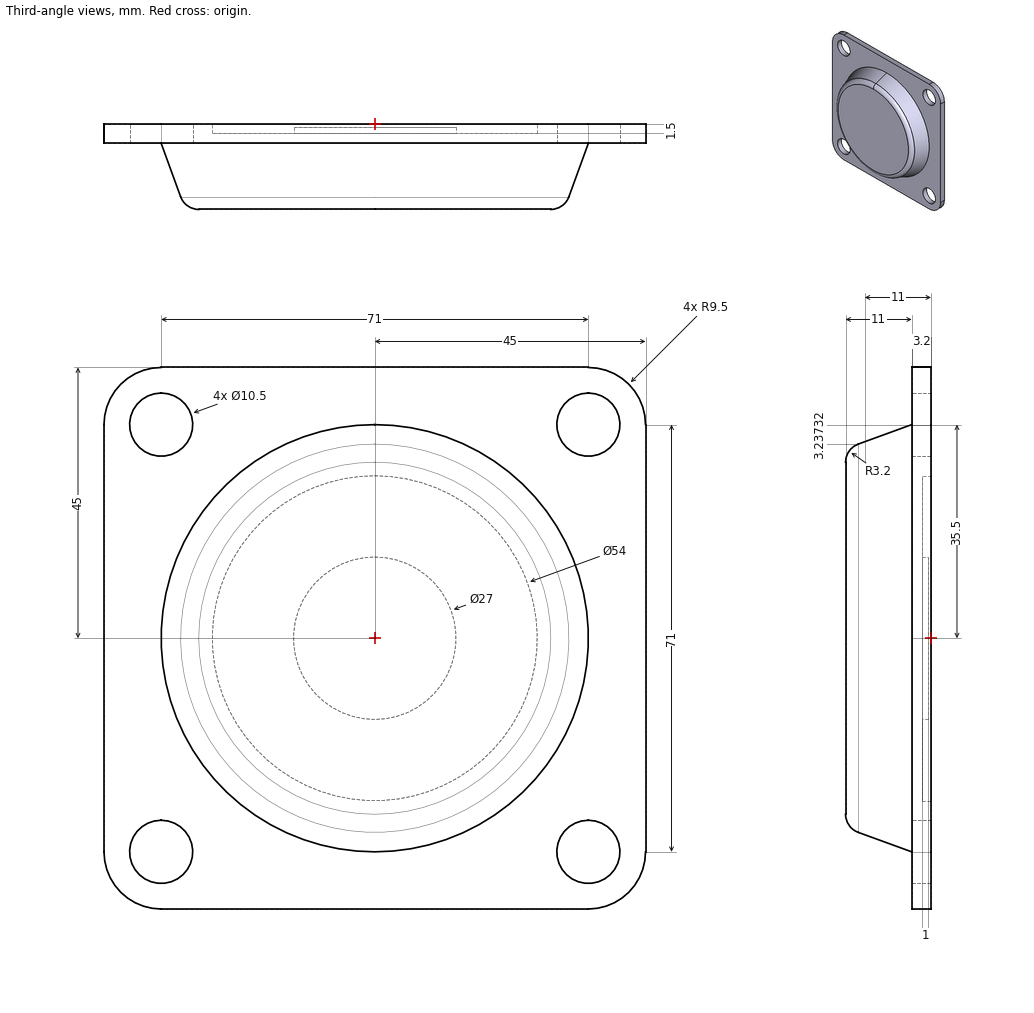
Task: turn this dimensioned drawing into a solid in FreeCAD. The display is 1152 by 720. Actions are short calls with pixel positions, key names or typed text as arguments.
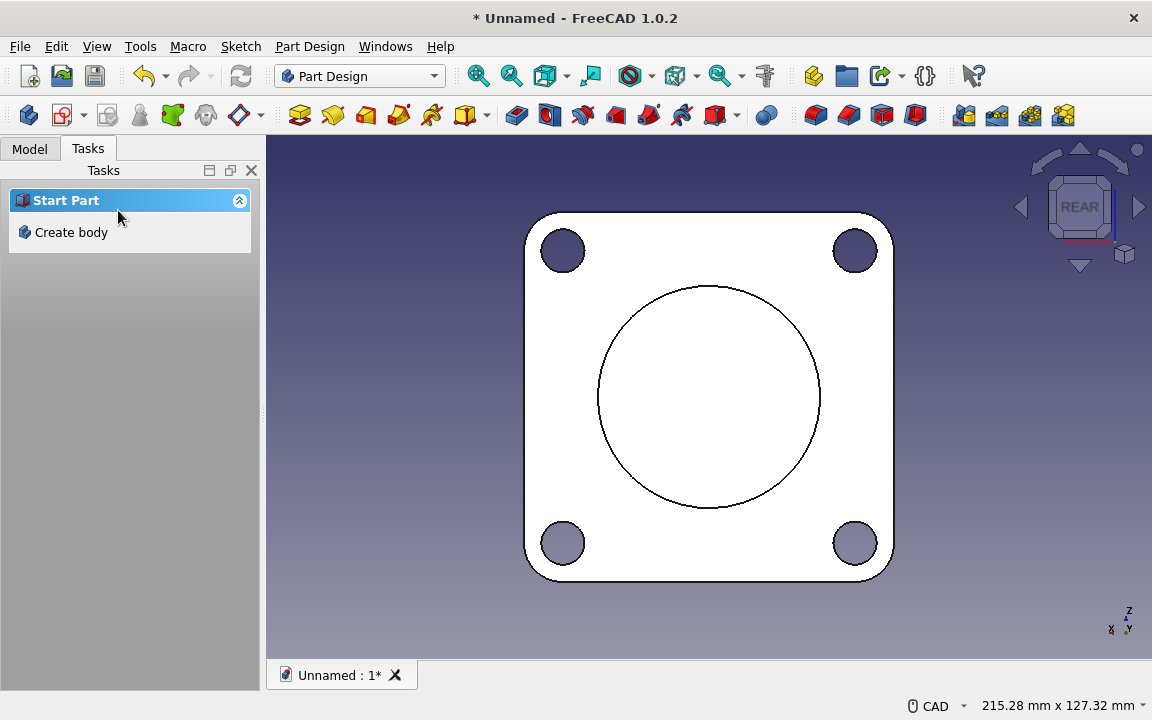
click(709, 396)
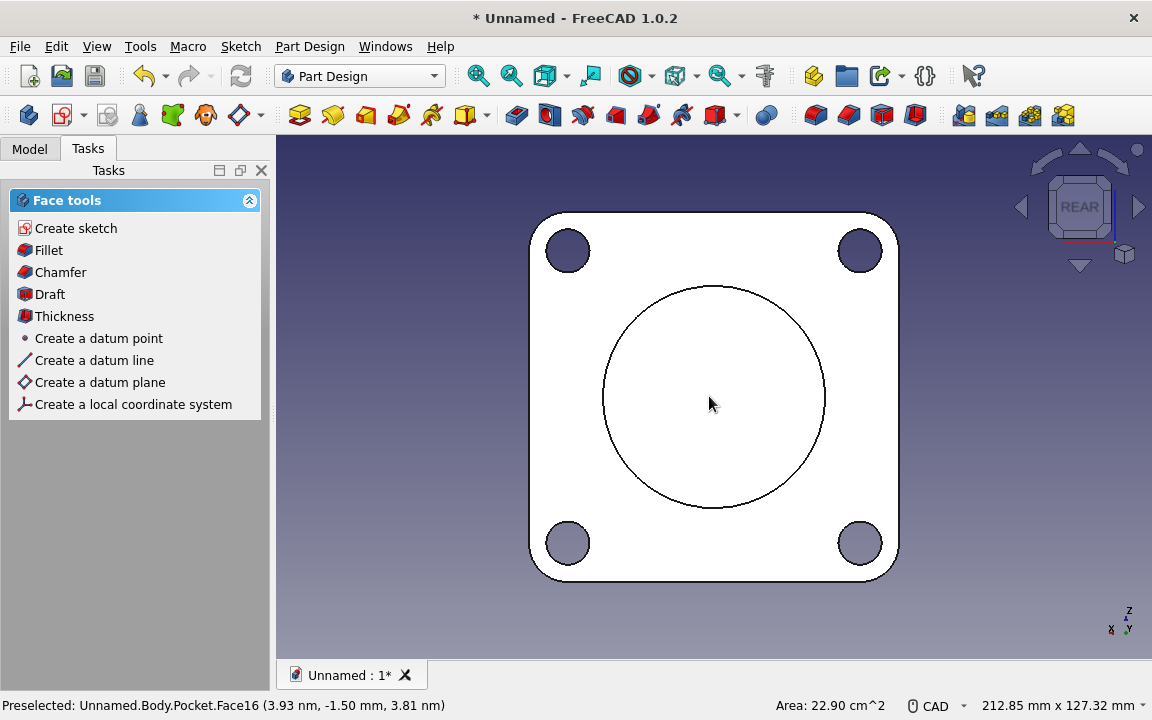
click(62, 116)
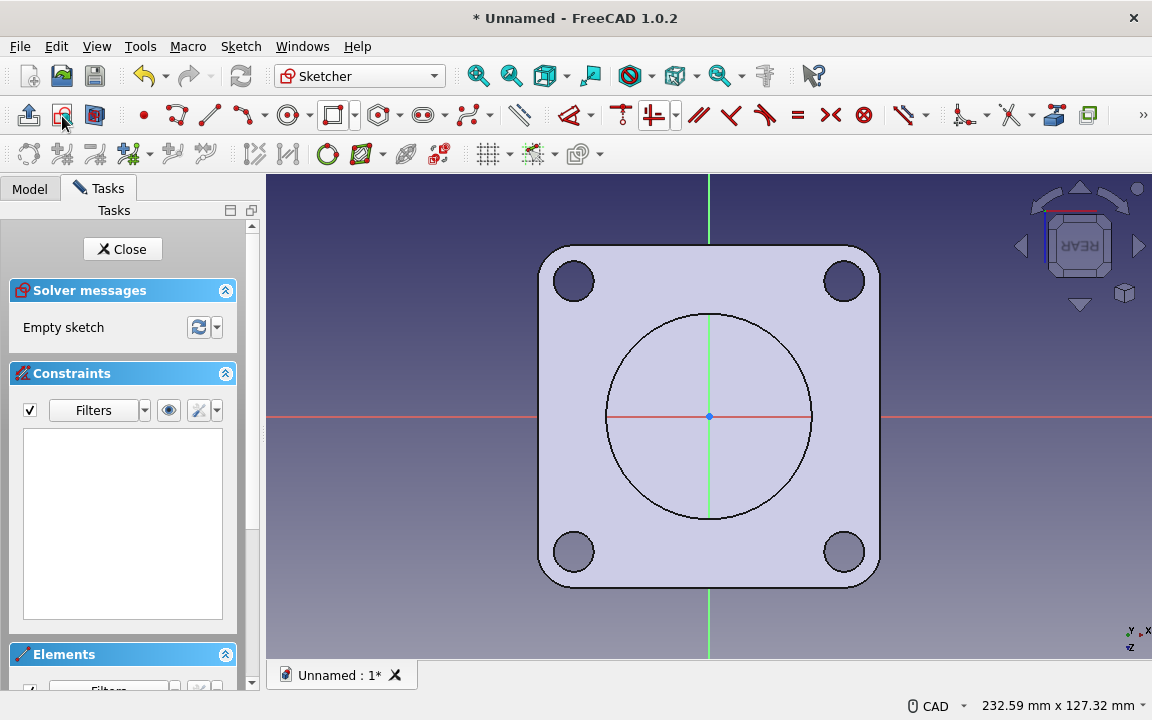
key(q)
key(s)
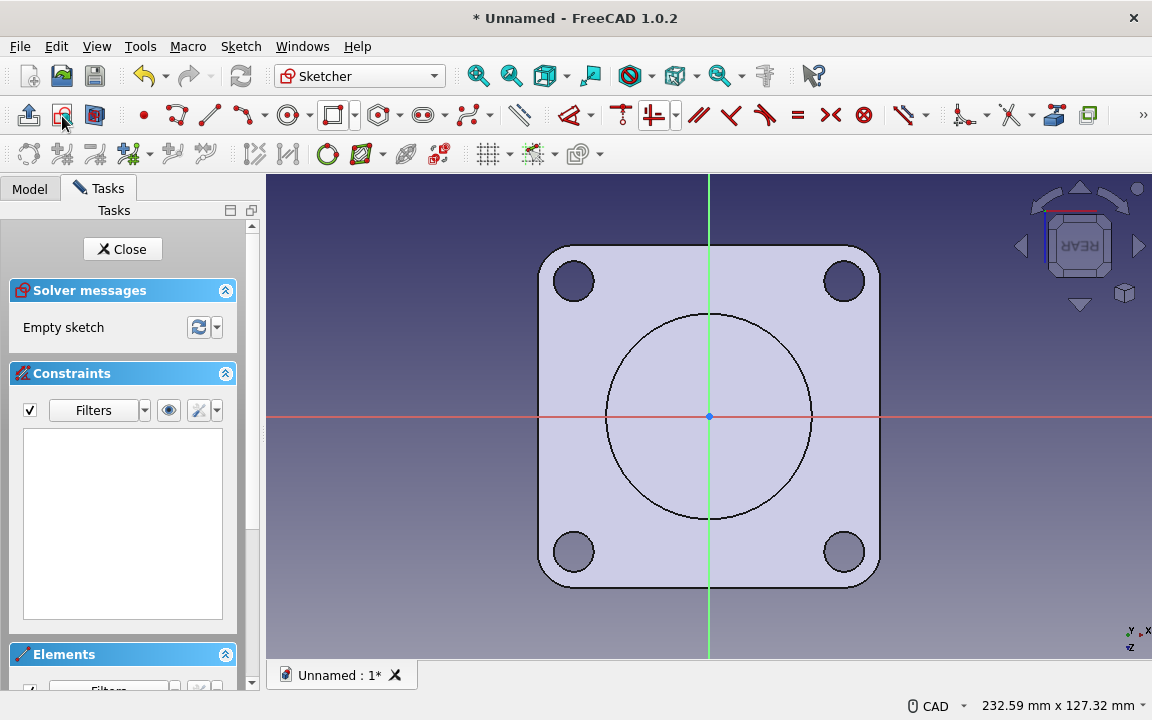
scroll(749, 416, up, 5)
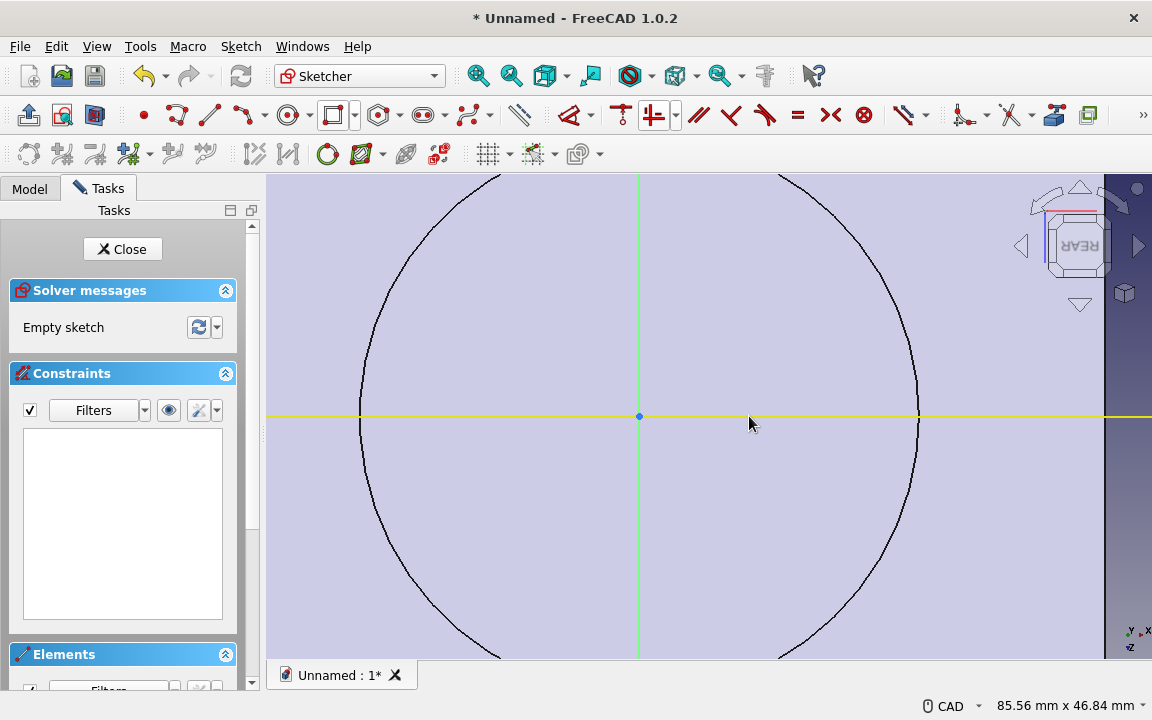
key(g)
key(c)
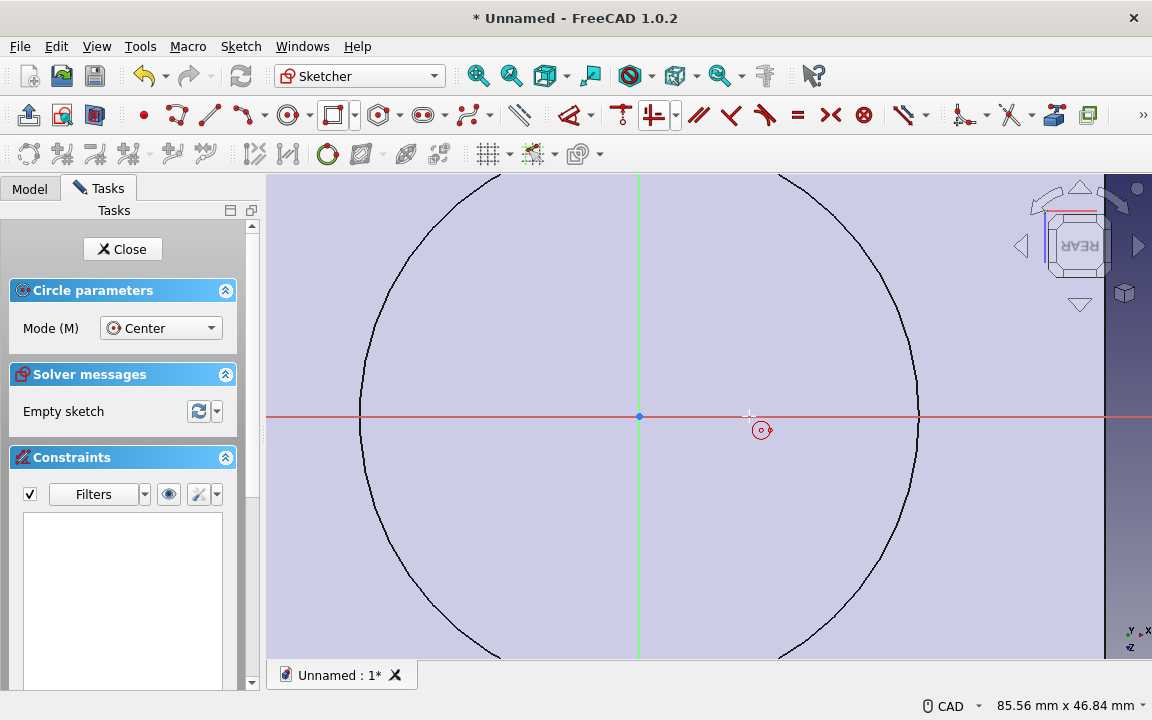
click(639, 416)
move(738, 318)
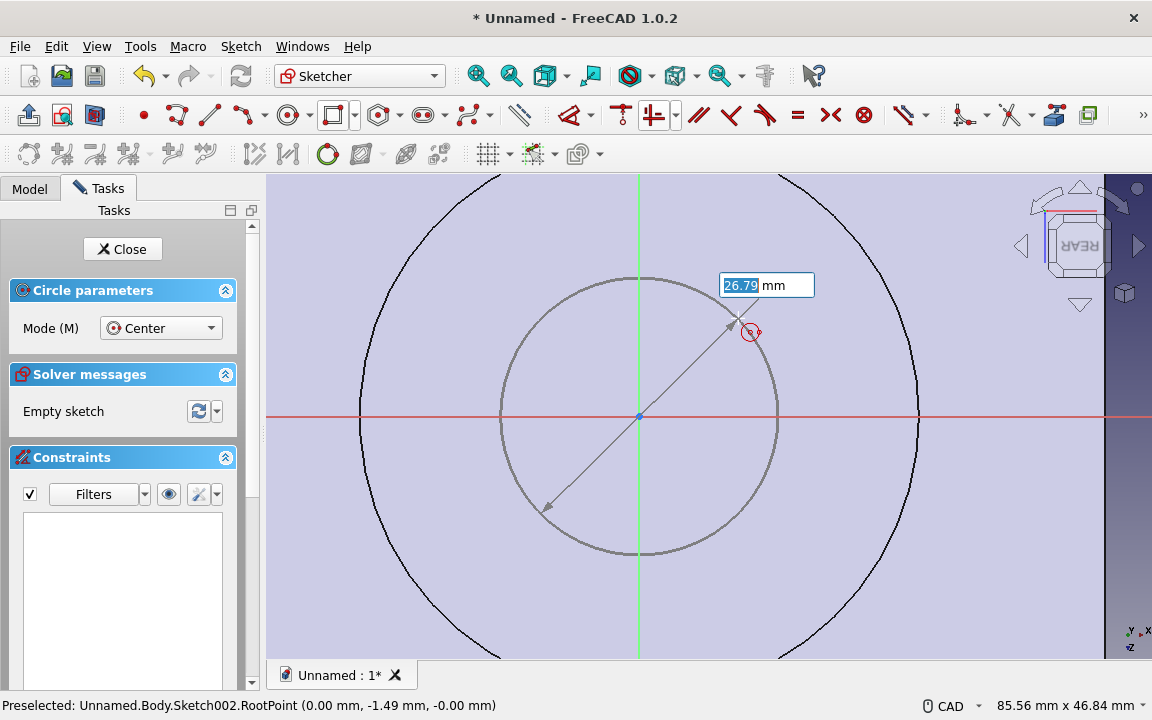
text(27)
key(Return)
key(Escape)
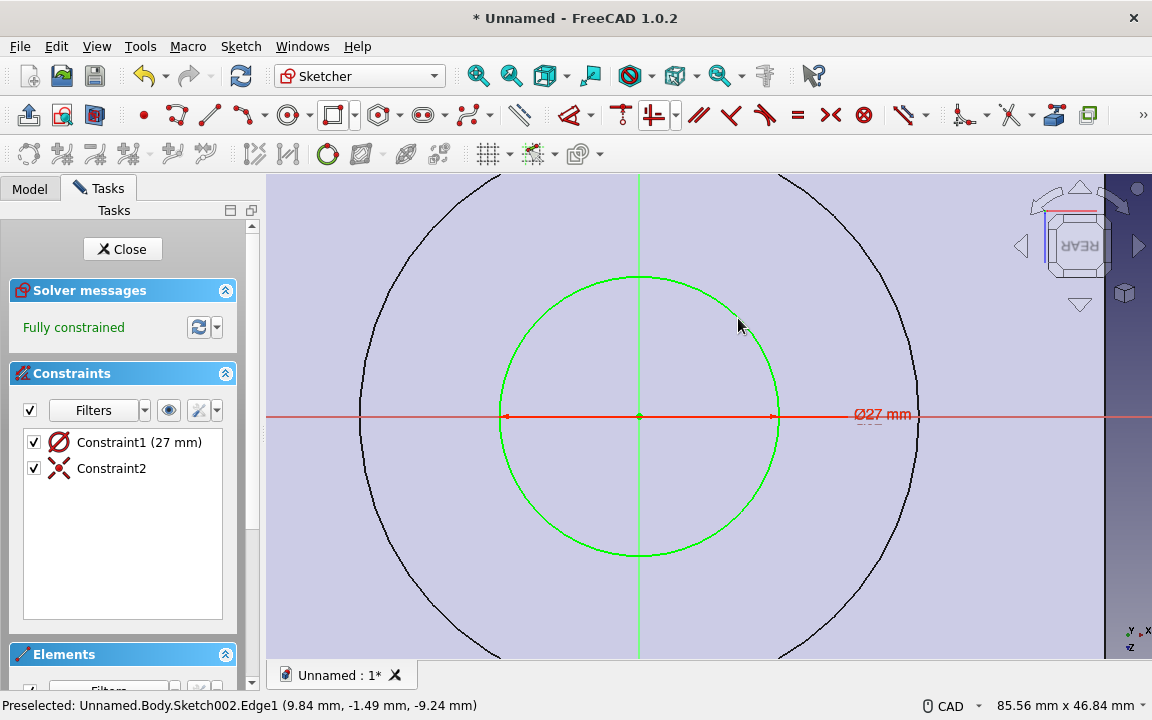
click(123, 249)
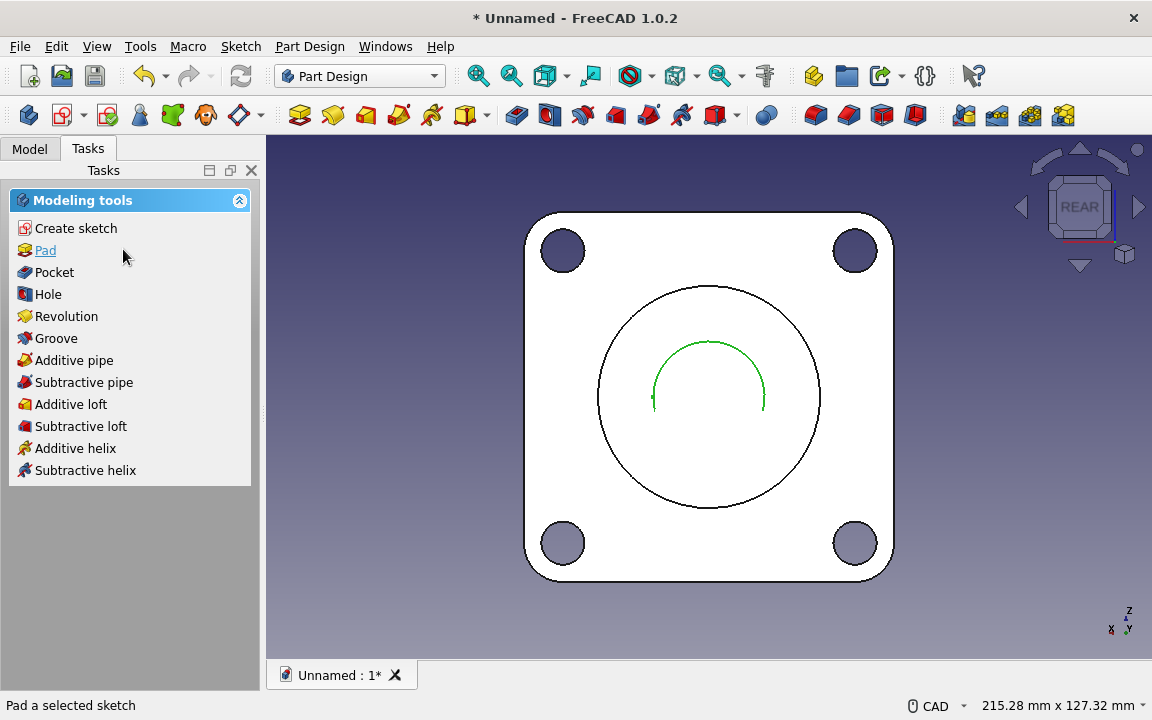
click(300, 116)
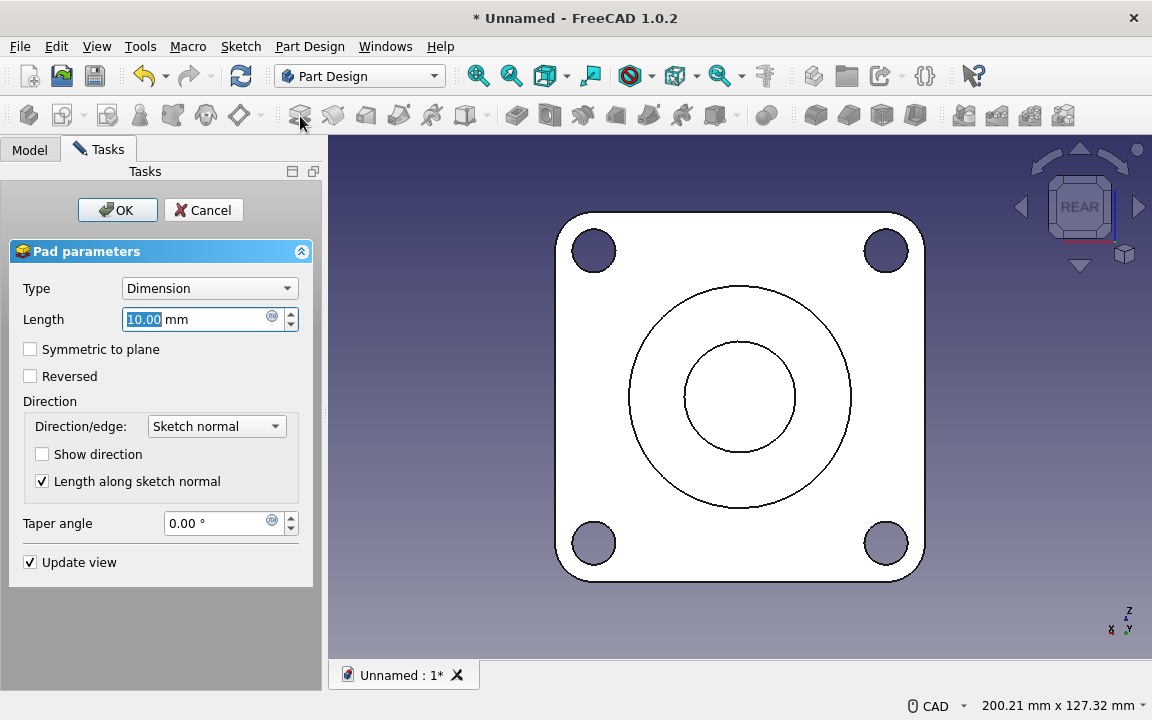
text(1)
key(Tab)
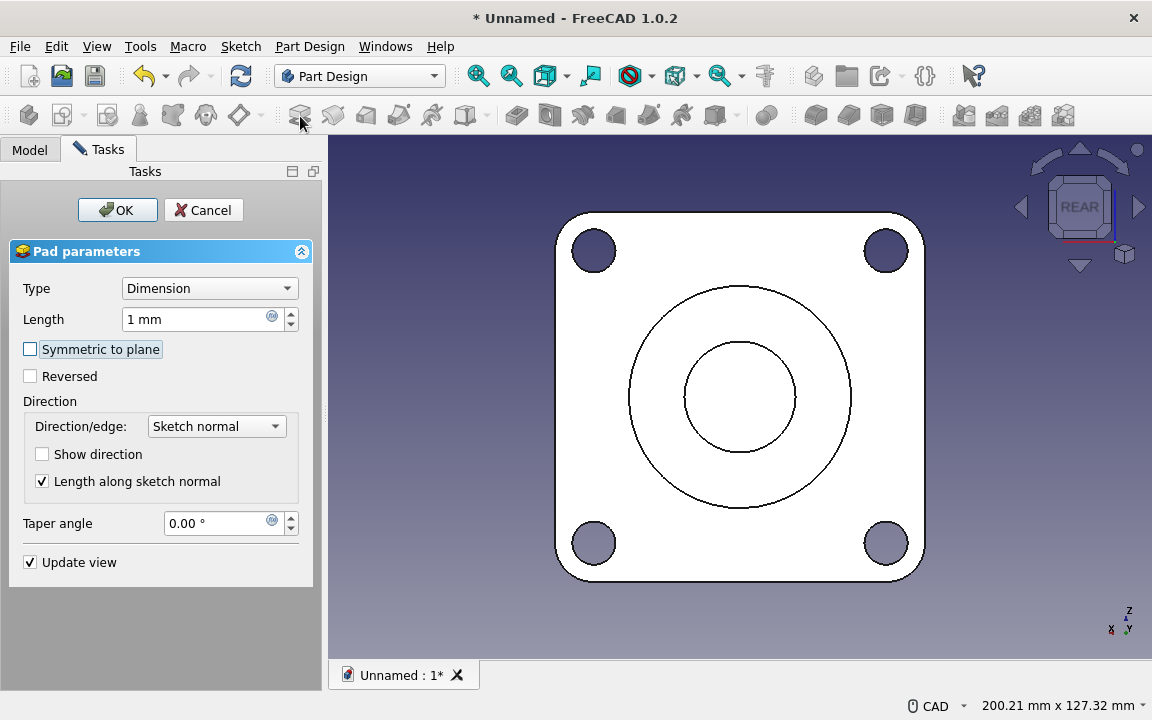
click(118, 210)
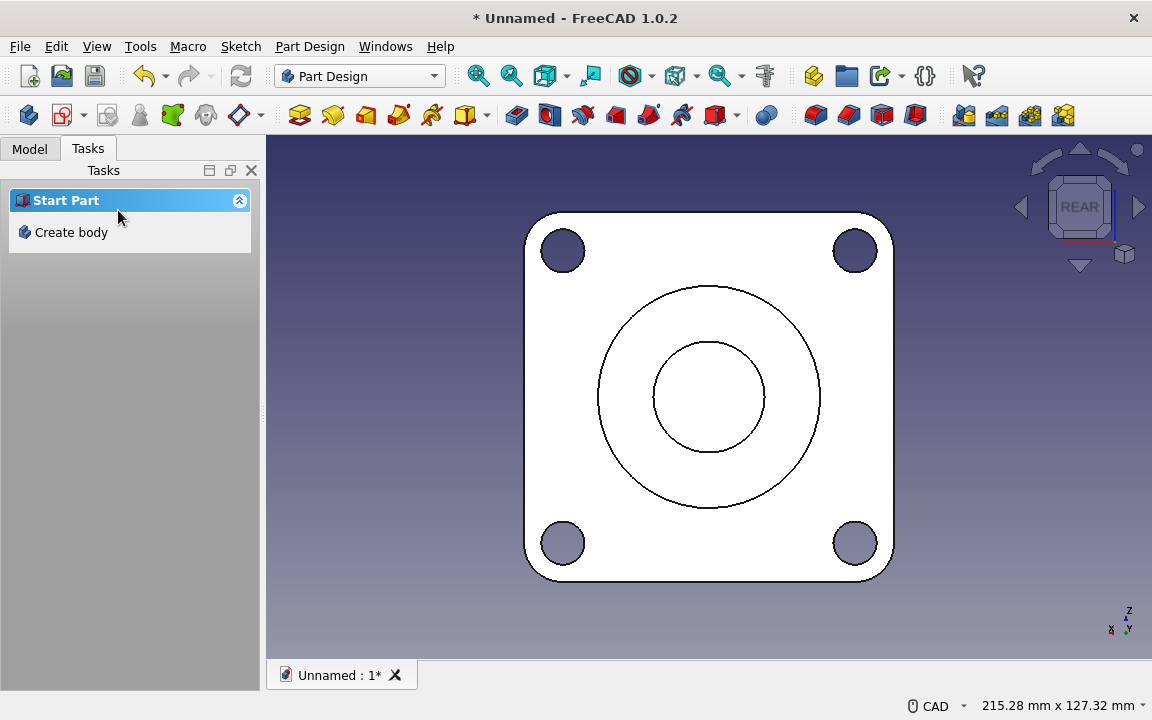
click(62, 116)